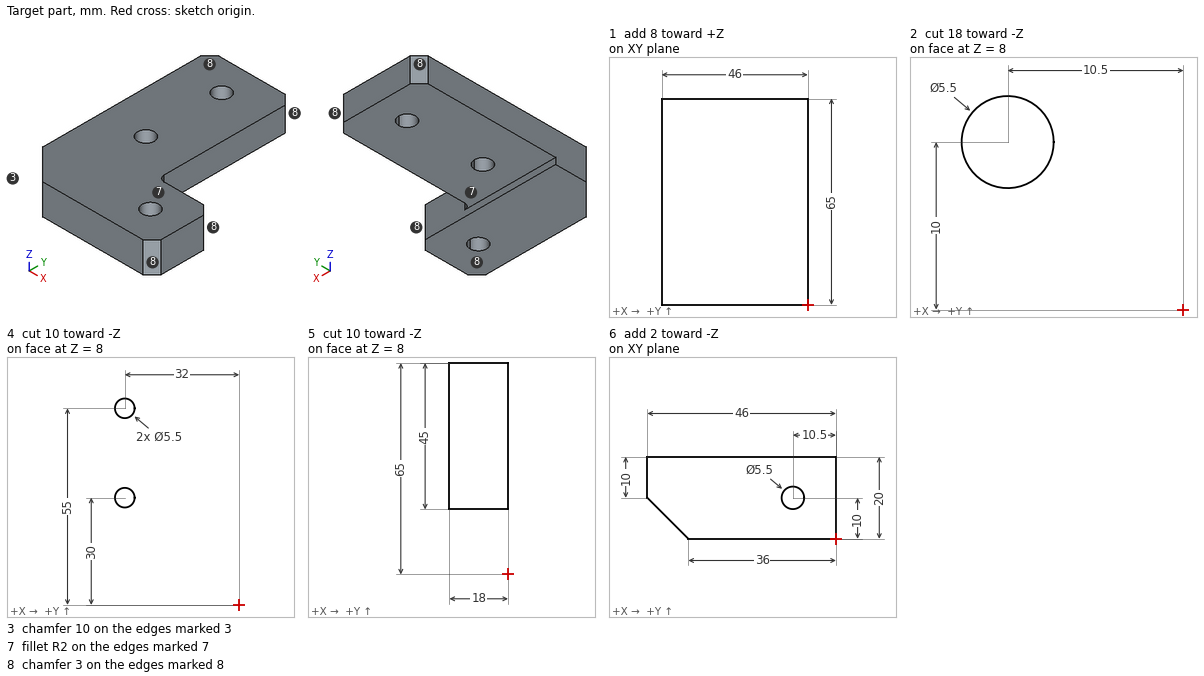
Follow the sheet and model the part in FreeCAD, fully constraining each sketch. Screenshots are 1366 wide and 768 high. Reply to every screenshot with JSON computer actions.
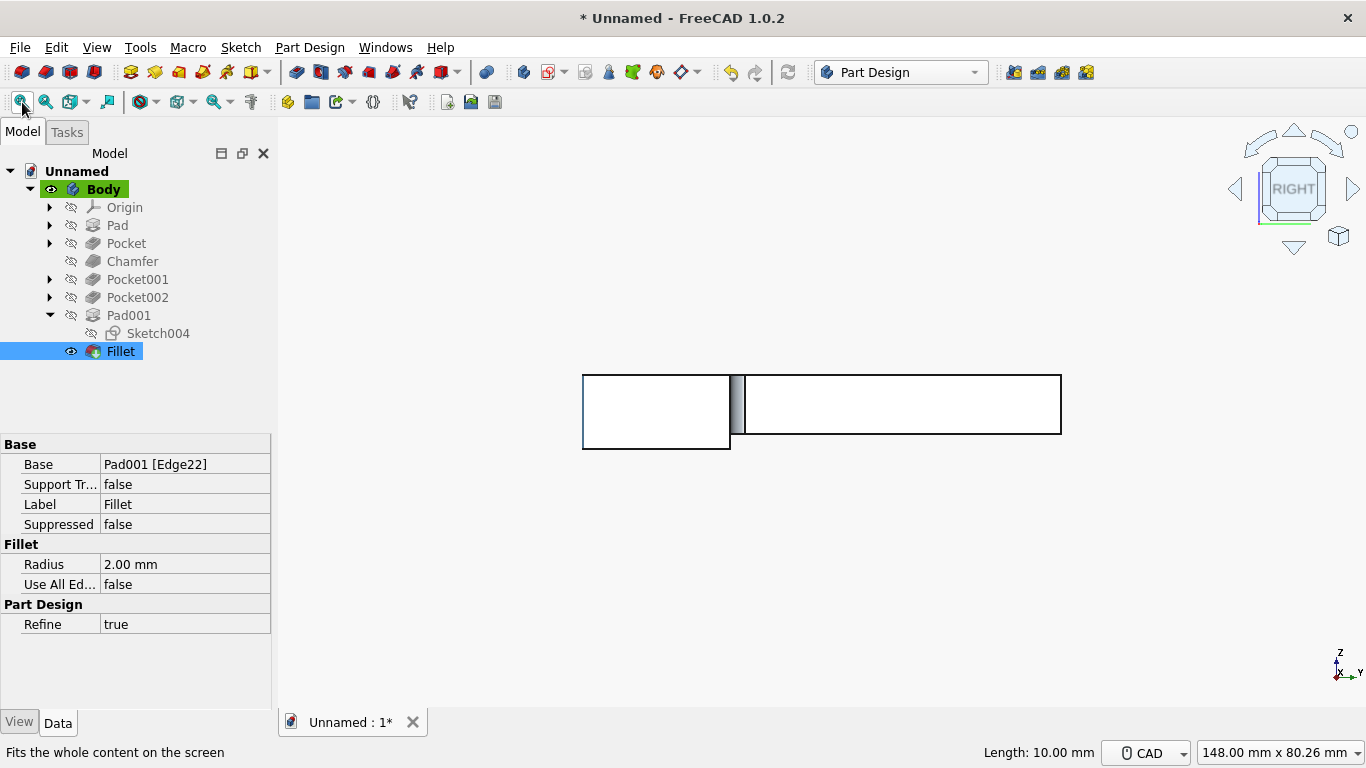
{"action": "left_click", "coordinate": [22, 102]}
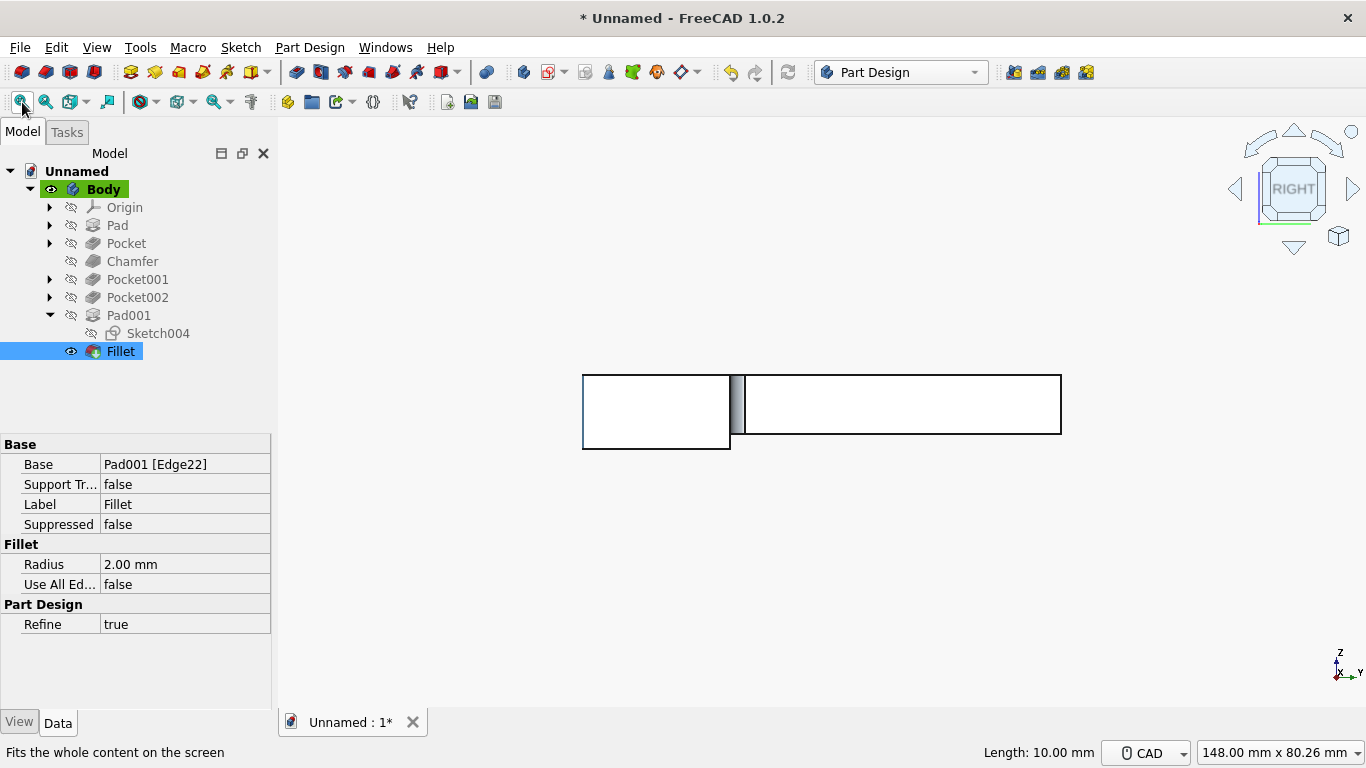
{"action": "left_click", "coordinate": [730, 411], "text": "ctrl"}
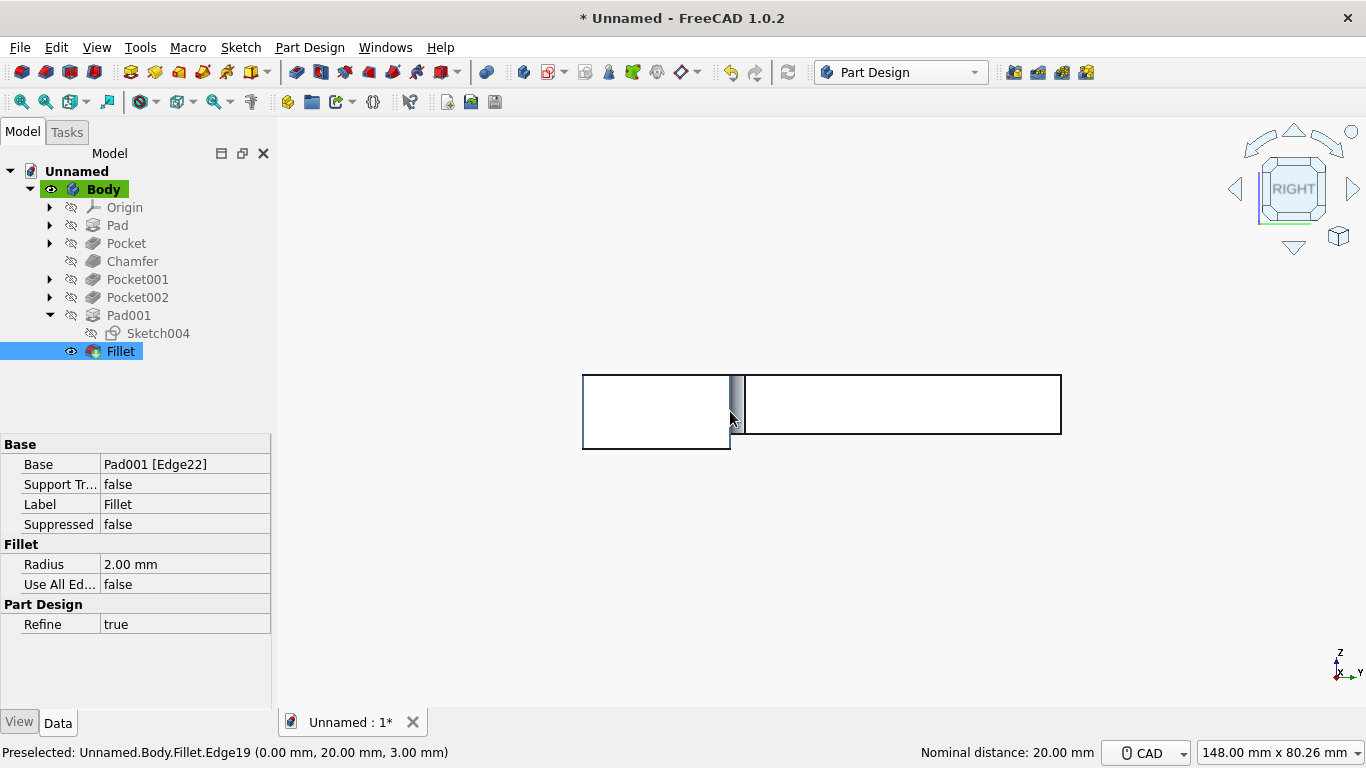
{"action": "left_click", "coordinate": [1061, 404], "text": "ctrl"}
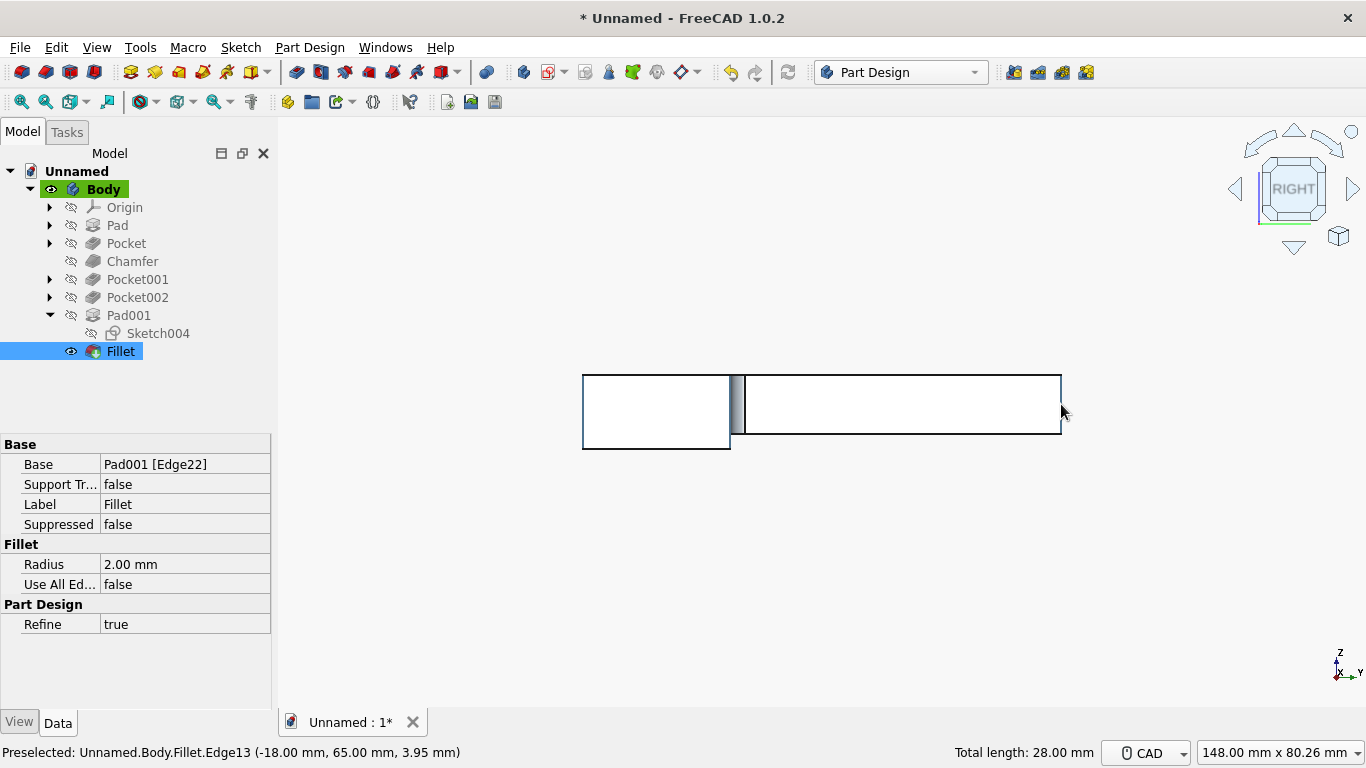
{"action": "key", "text": "5"}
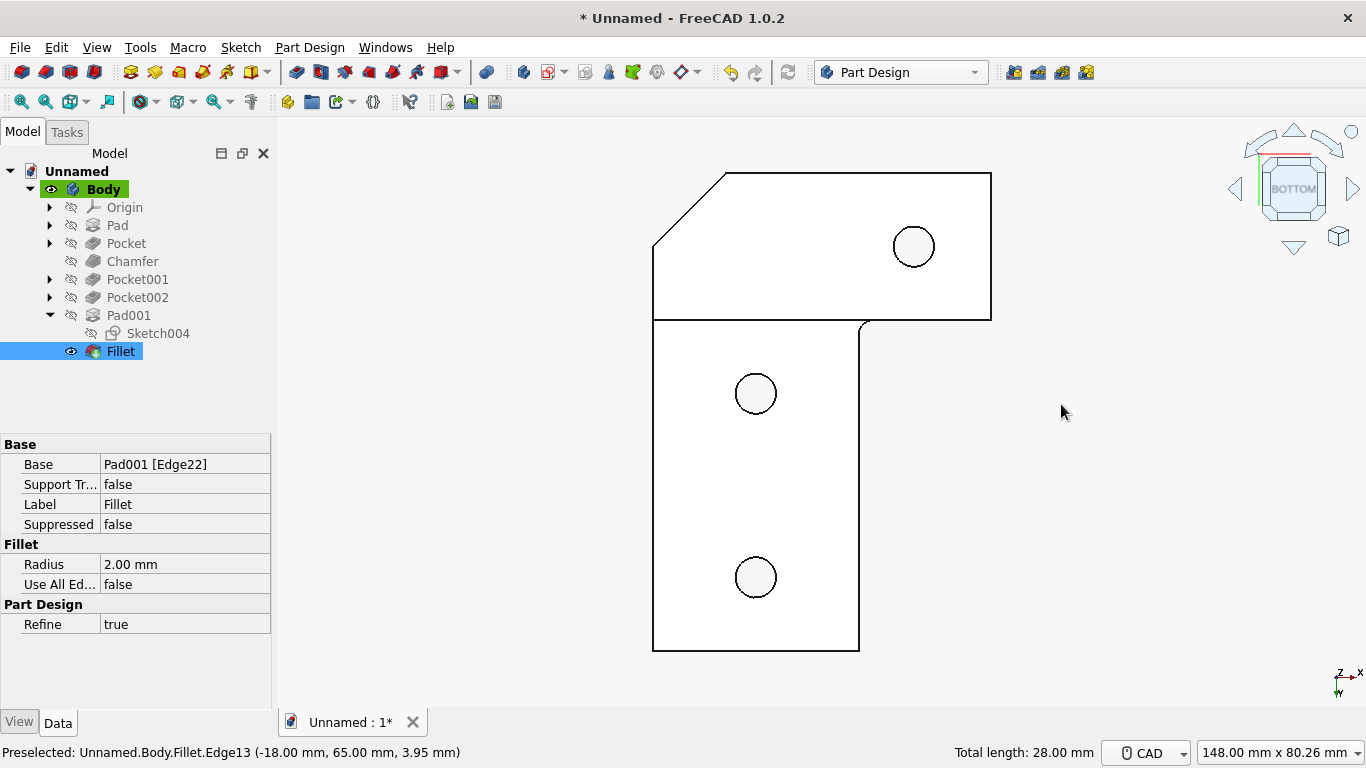
{"action": "key", "text": "4"}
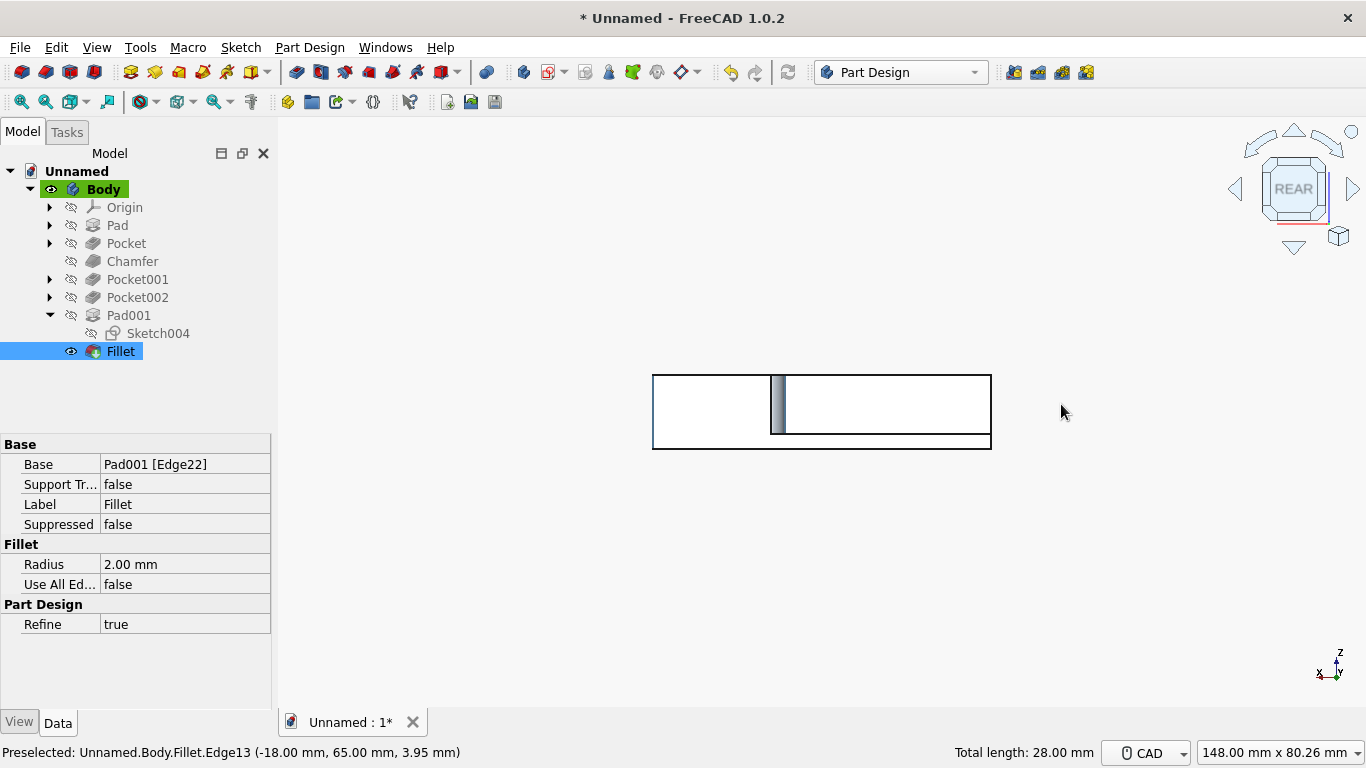
{"action": "left_click", "coordinate": [22, 102]}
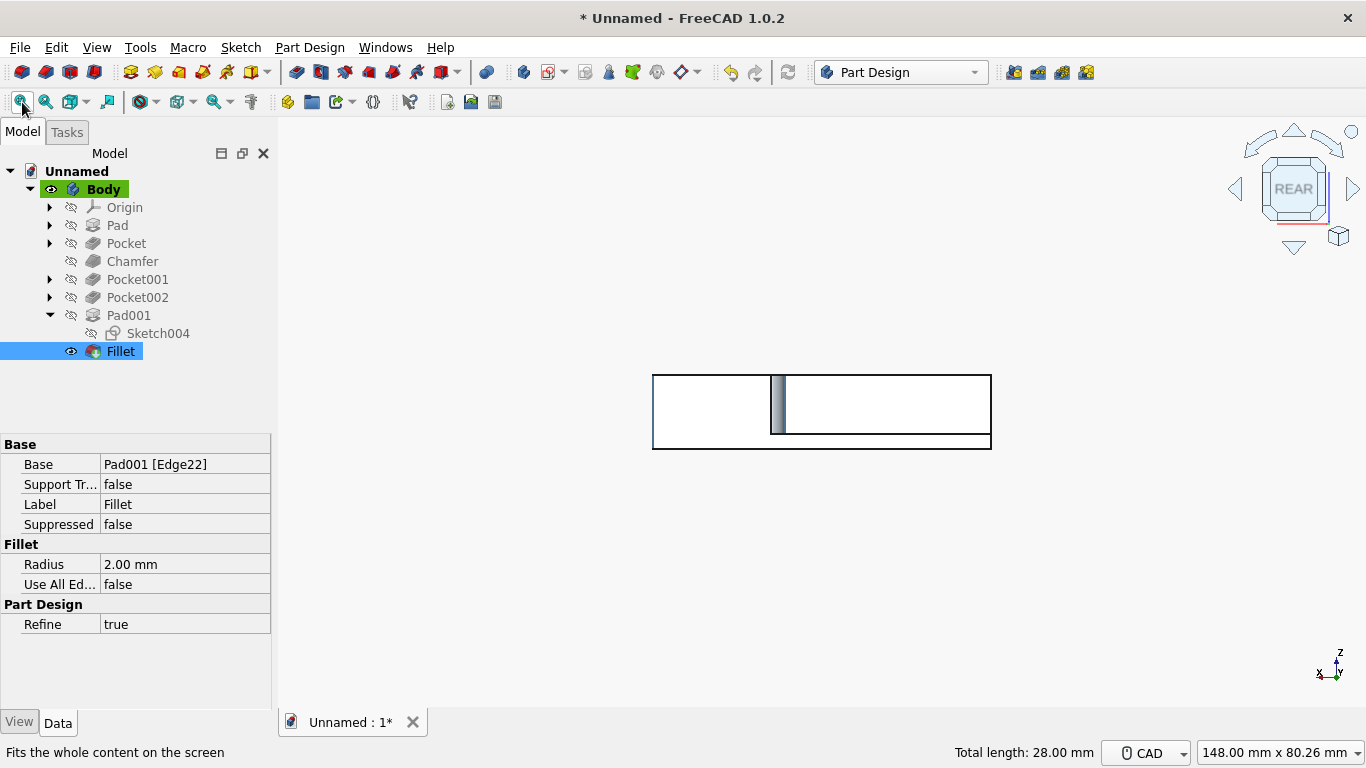
{"action": "left_click", "coordinate": [991, 404], "text": "ctrl"}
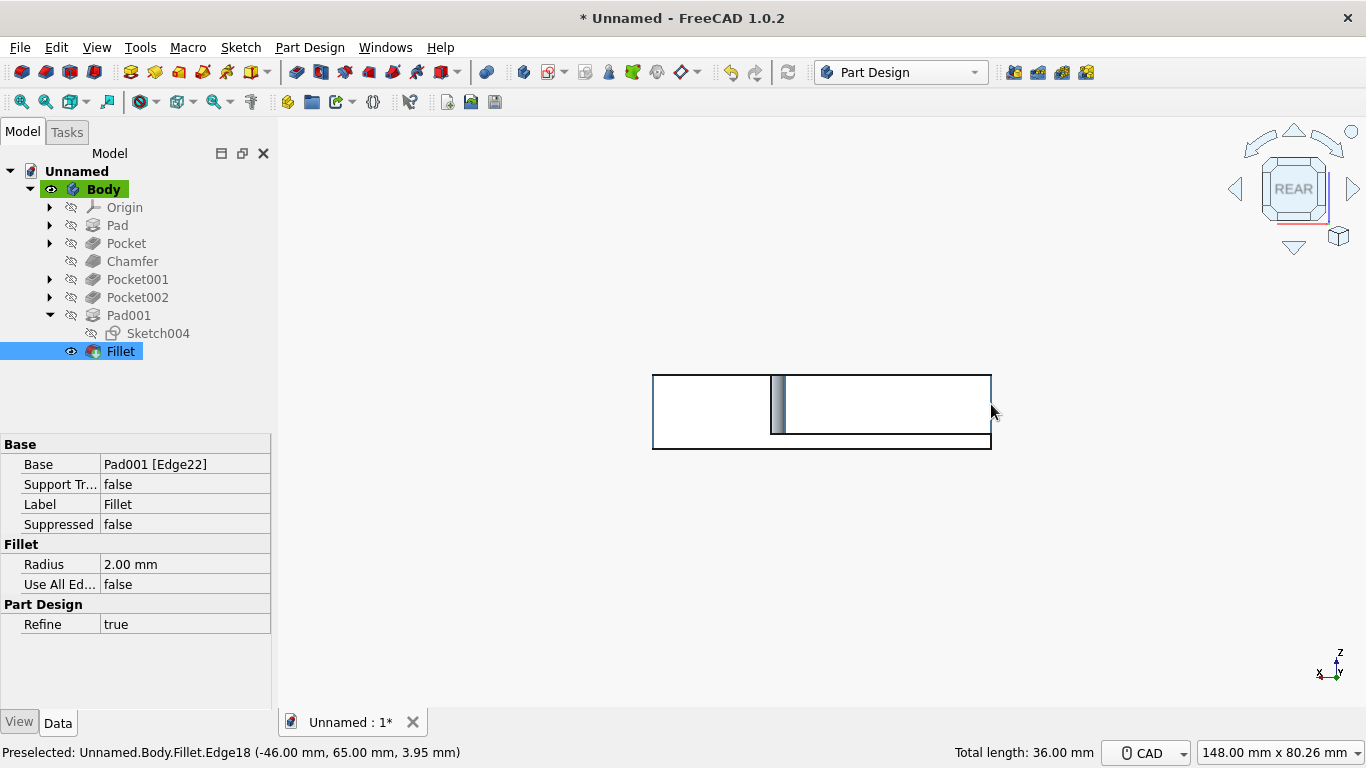
{"action": "left_click", "coordinate": [46, 72]}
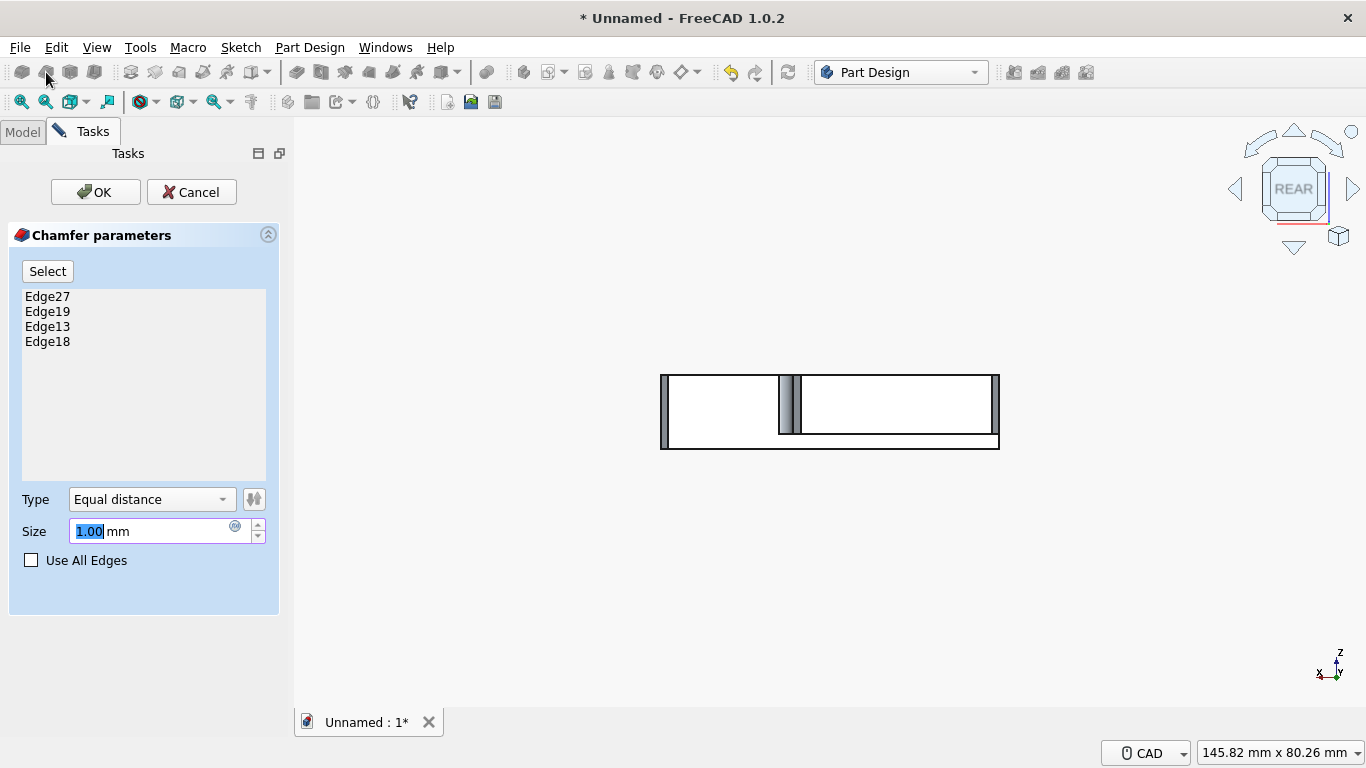
{"action": "type", "text": "3"}
{"action": "key", "text": "Tab"}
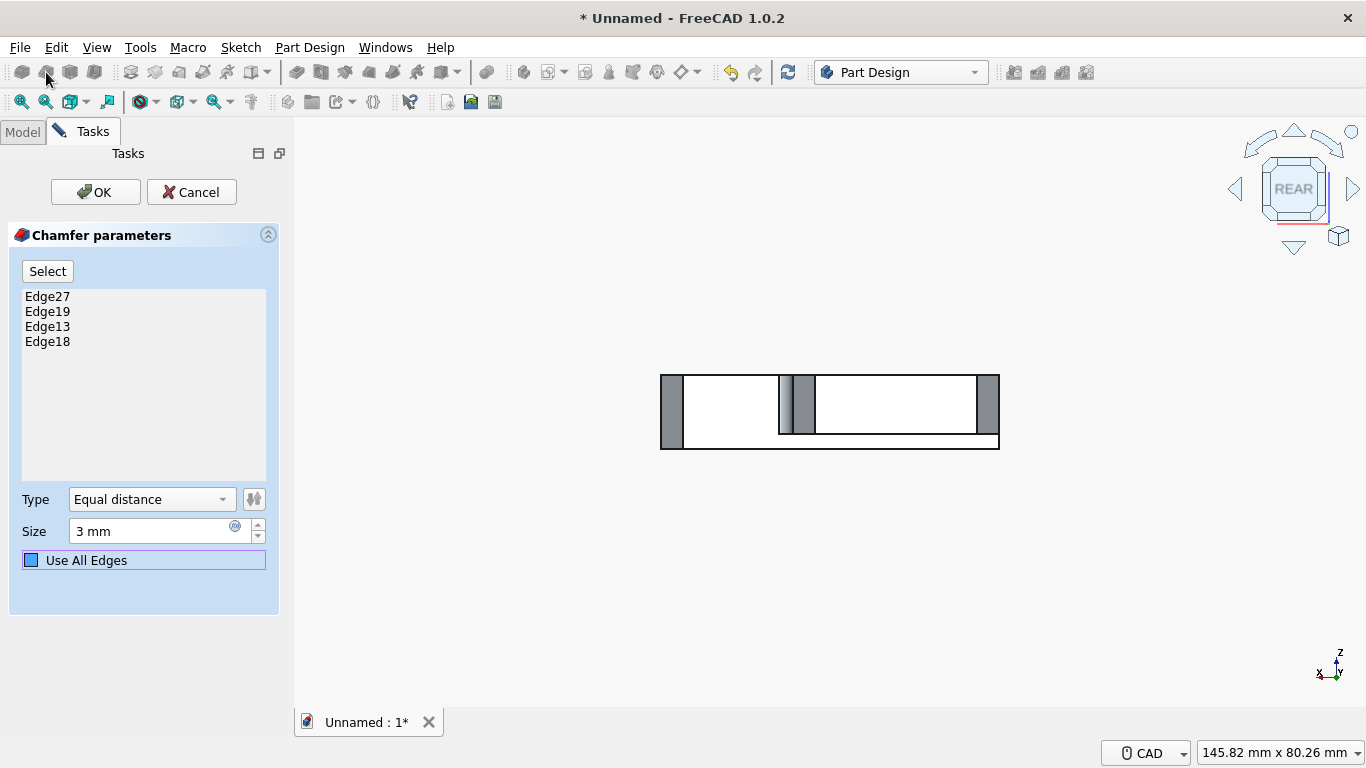
{"action": "left_click", "coordinate": [96, 192]}